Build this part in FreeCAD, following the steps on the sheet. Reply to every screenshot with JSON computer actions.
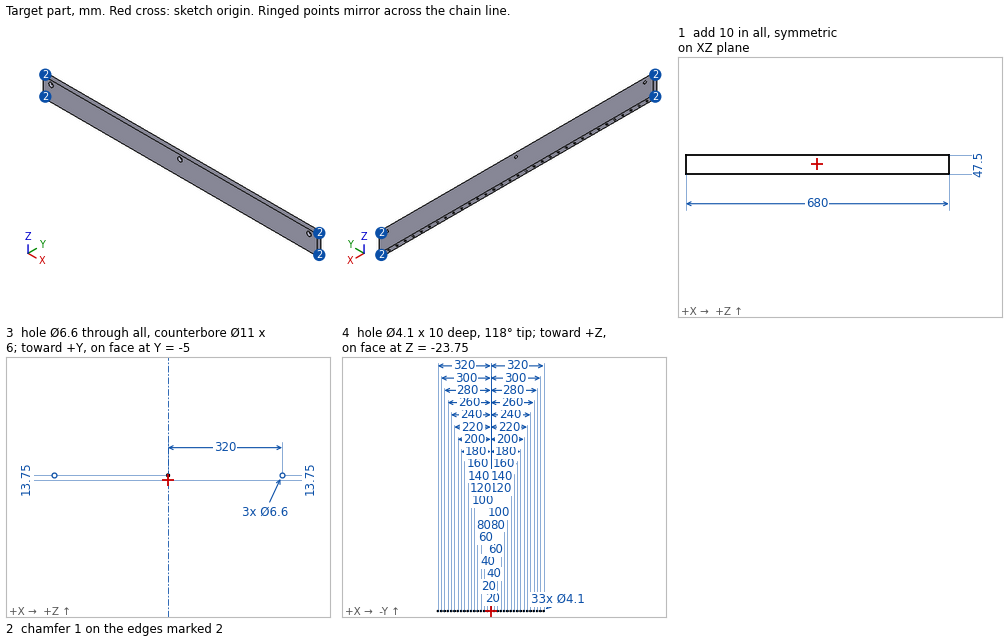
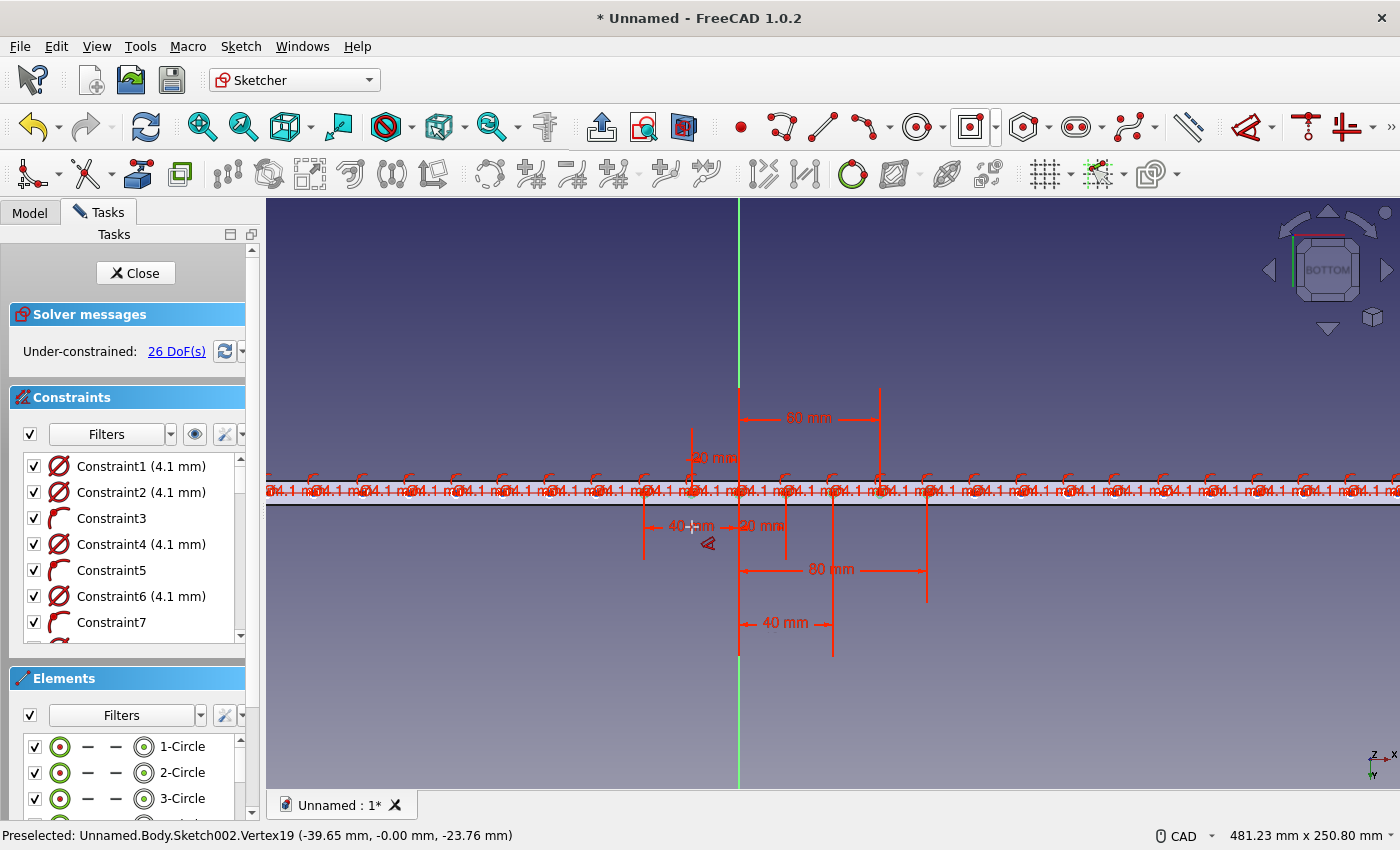
{"action": "left_click", "coordinate": [596, 493]}
{"action": "left_click", "coordinate": [618, 527]}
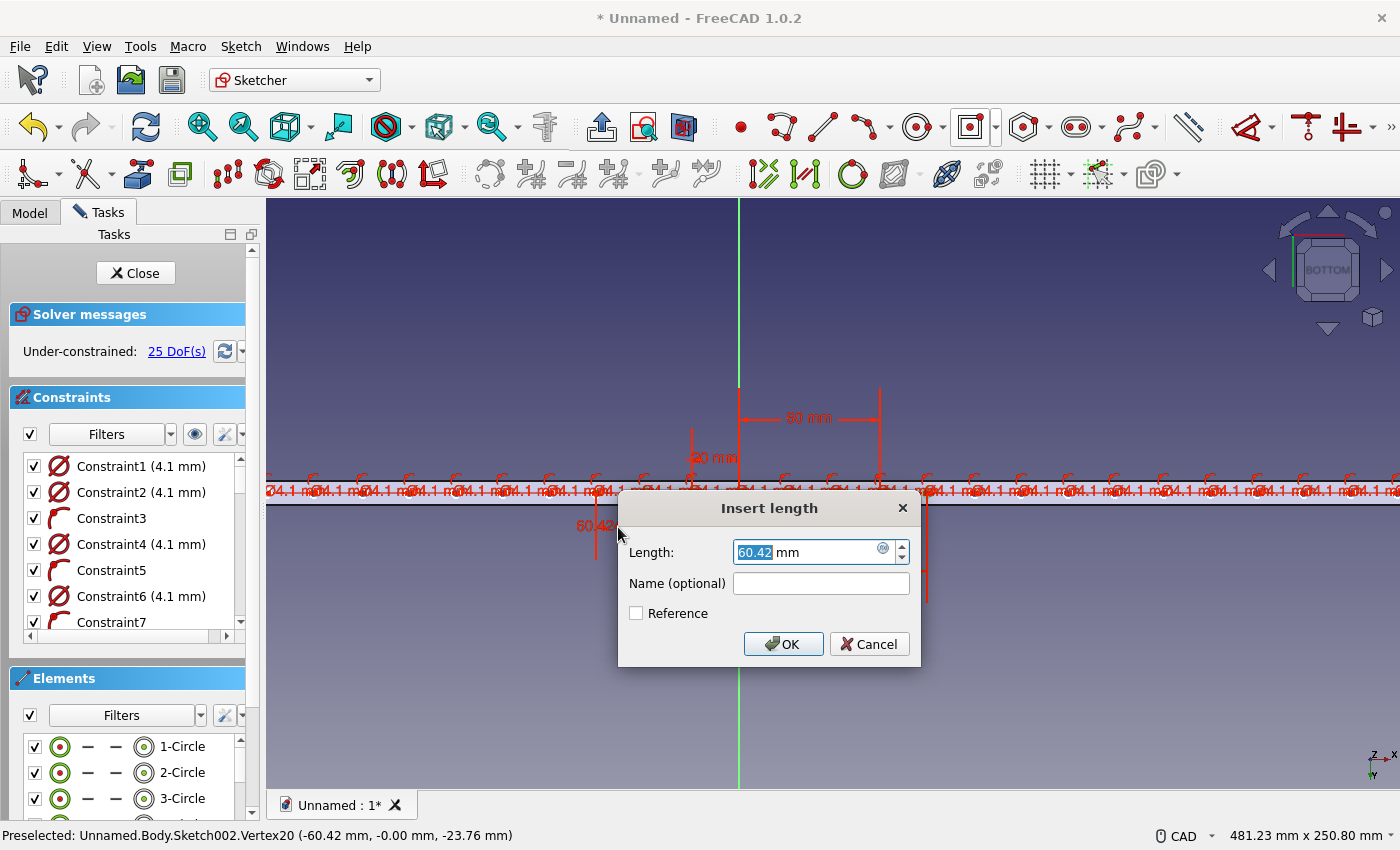
{"action": "type", "text": "60"}
{"action": "key", "text": "Return"}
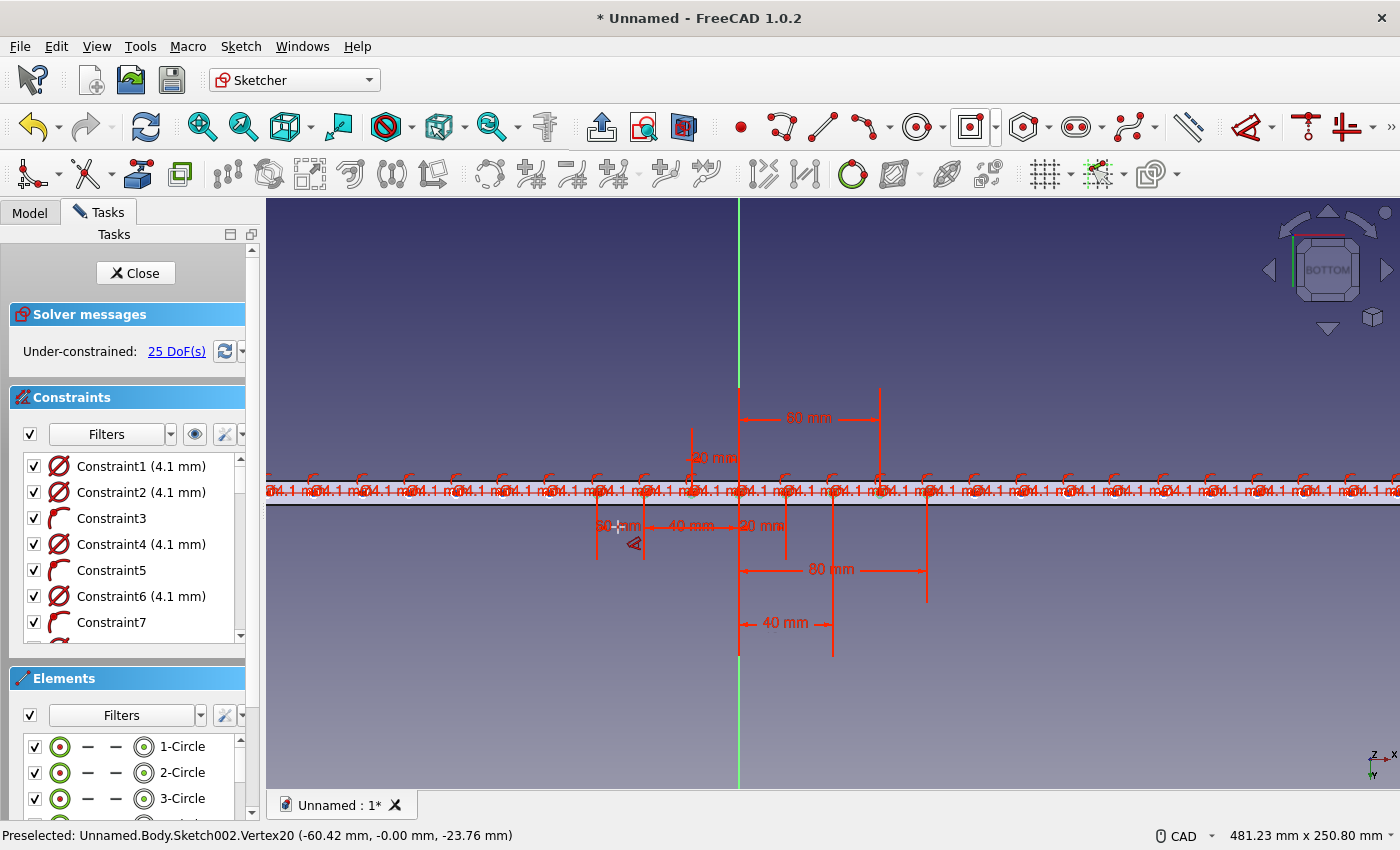
{"action": "left_click", "coordinate": [550, 493]}
{"action": "left_click", "coordinate": [644, 459]}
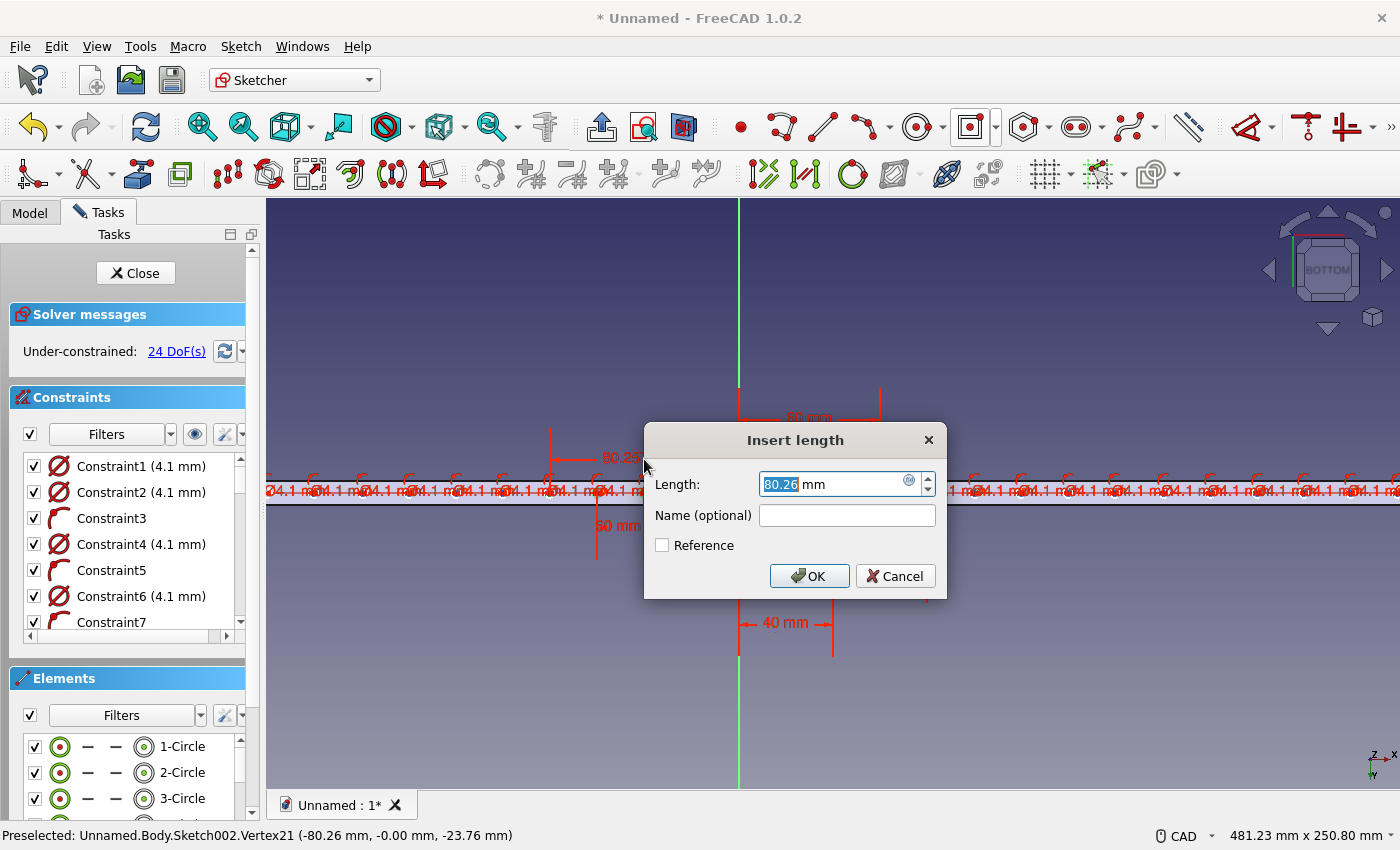
{"action": "type", "text": "80"}
{"action": "key", "text": "Return"}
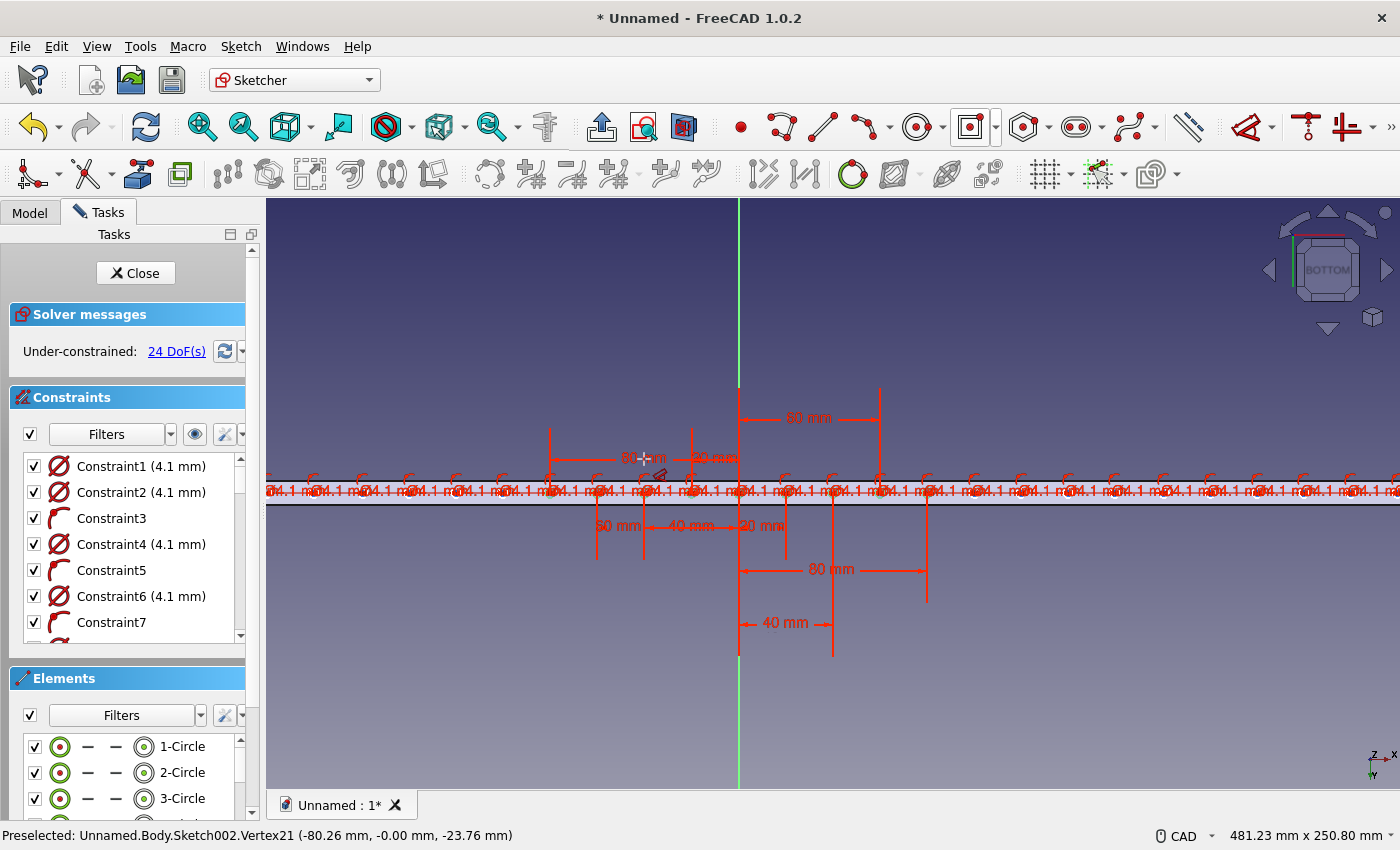
{"action": "scroll", "coordinate": [786, 494], "scroll_direction": "down", "scroll_amount": 4}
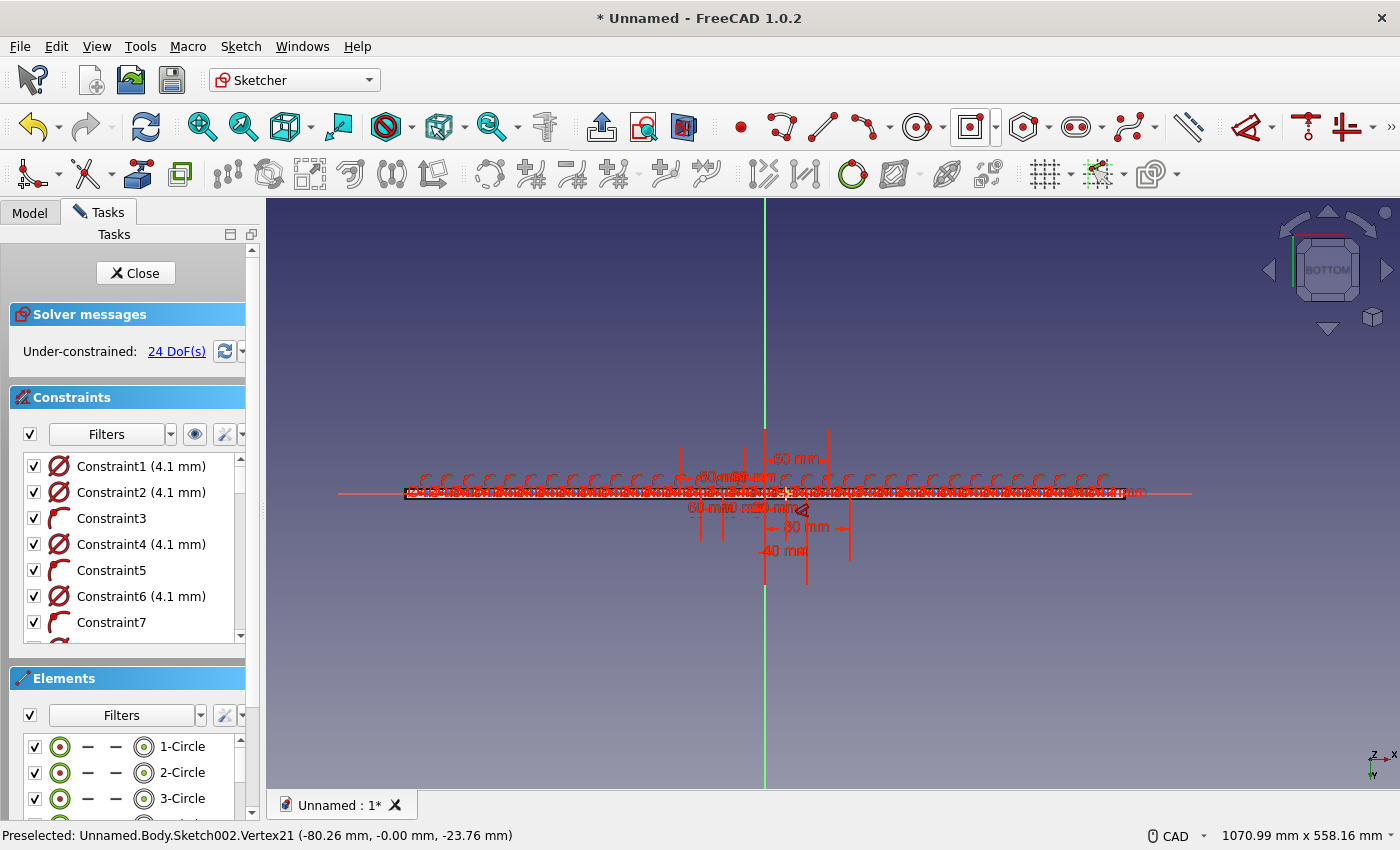
{"action": "left_click", "coordinate": [1104, 494]}
{"action": "left_click", "coordinate": [934, 528]}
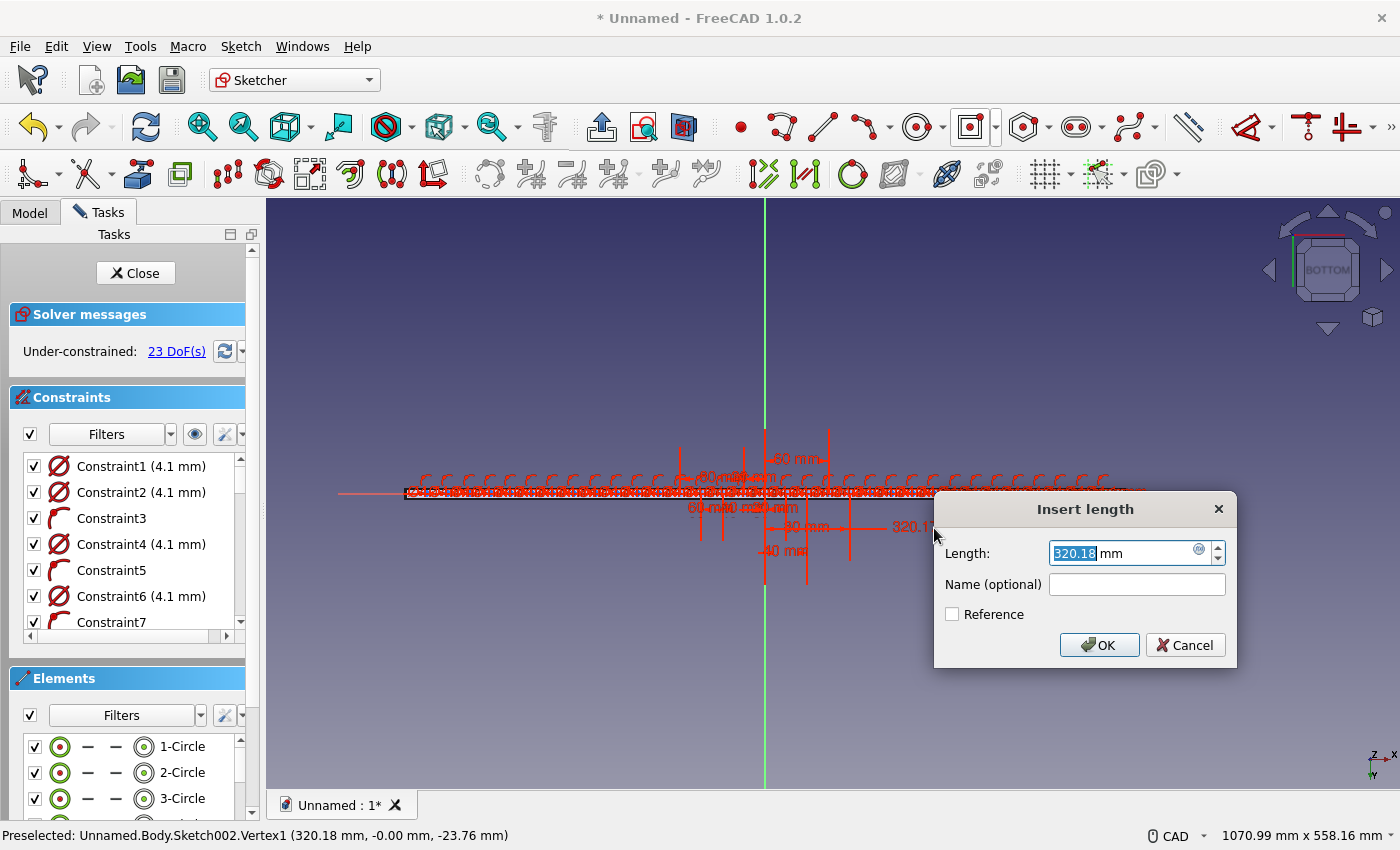
{"action": "type", "text": "320"}
{"action": "key", "text": "Return"}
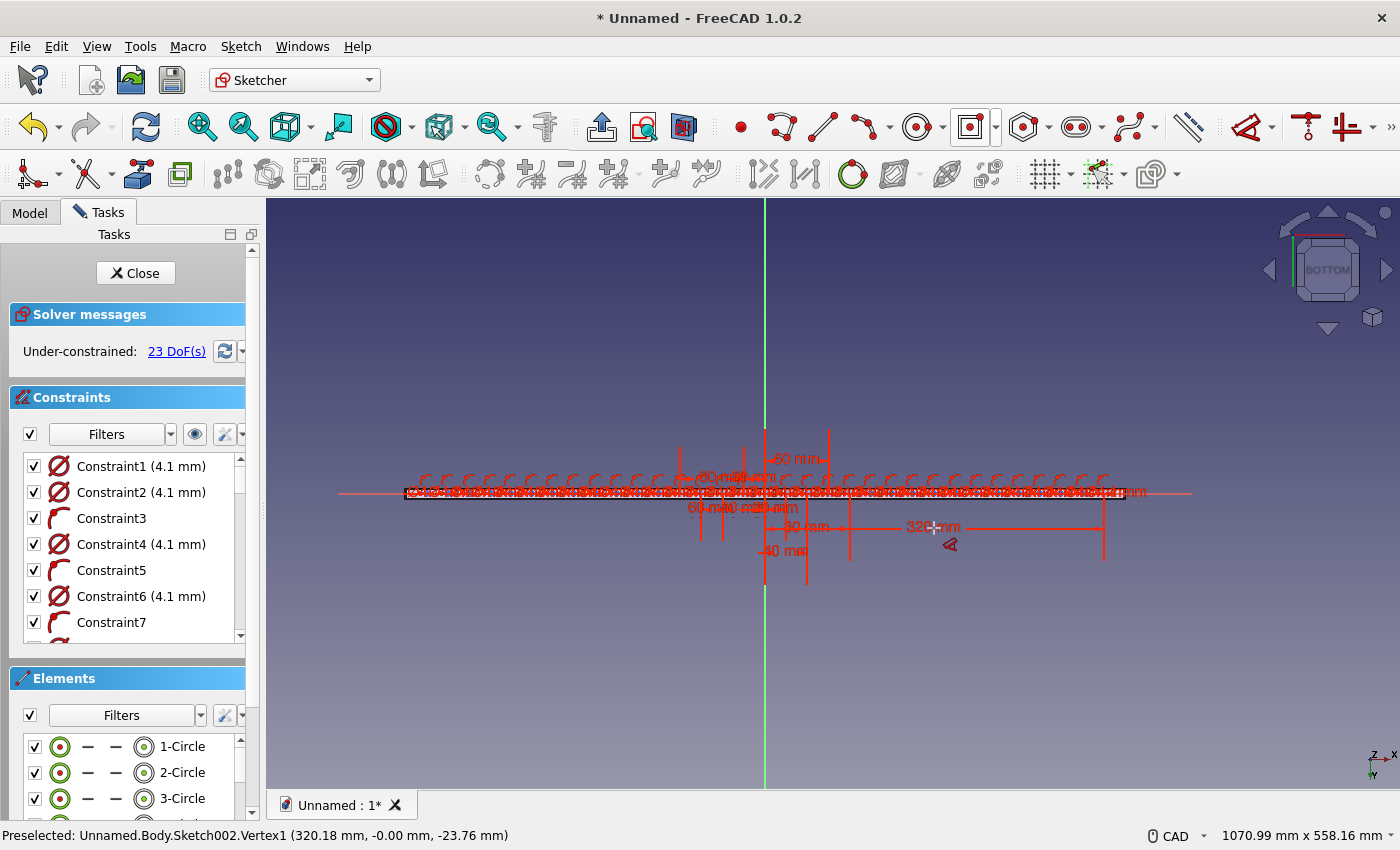
{"action": "left_click", "coordinate": [1083, 494]}
{"action": "left_click", "coordinate": [1035, 528]}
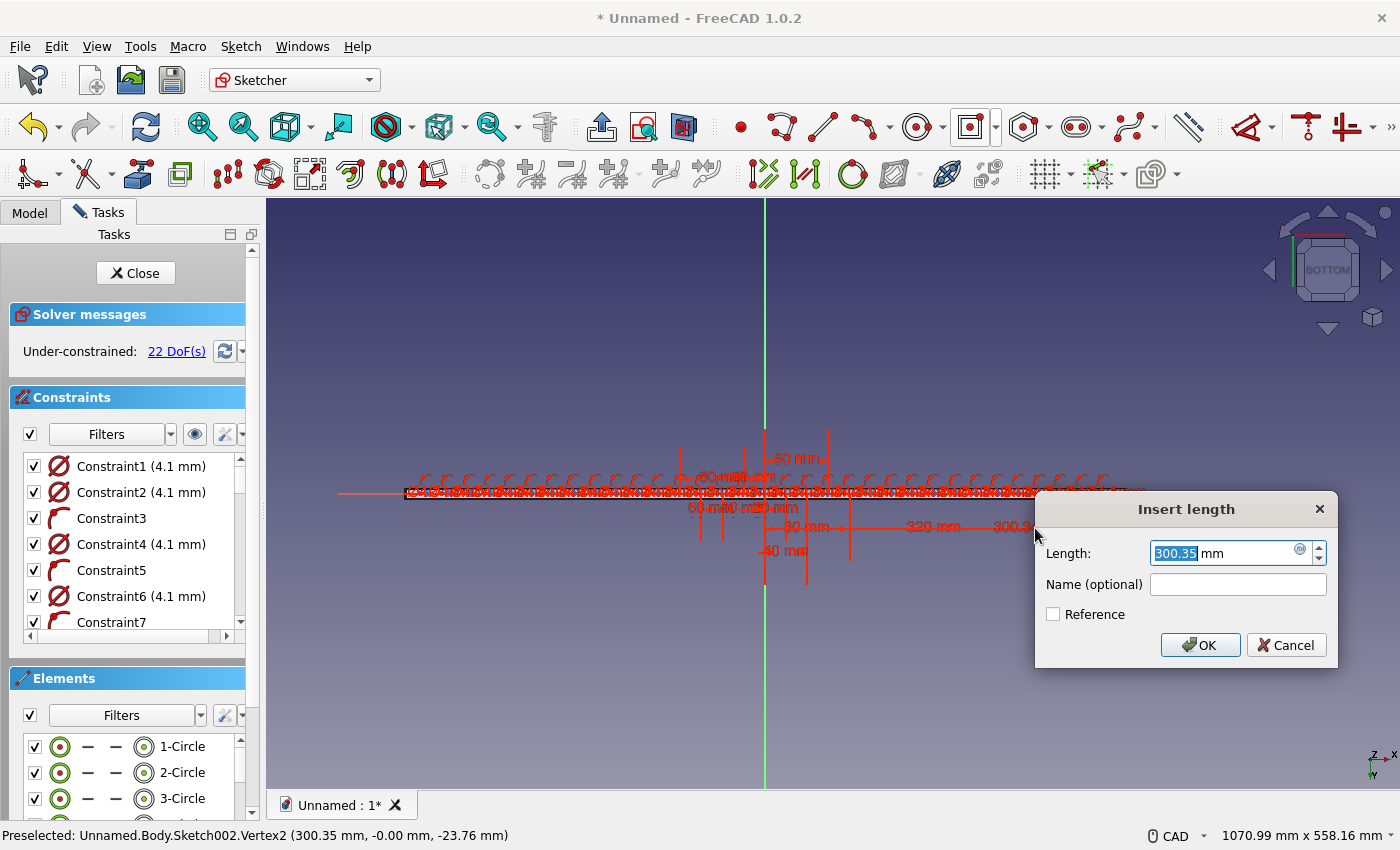
{"action": "type", "text": "300"}
{"action": "key", "text": "Return"}